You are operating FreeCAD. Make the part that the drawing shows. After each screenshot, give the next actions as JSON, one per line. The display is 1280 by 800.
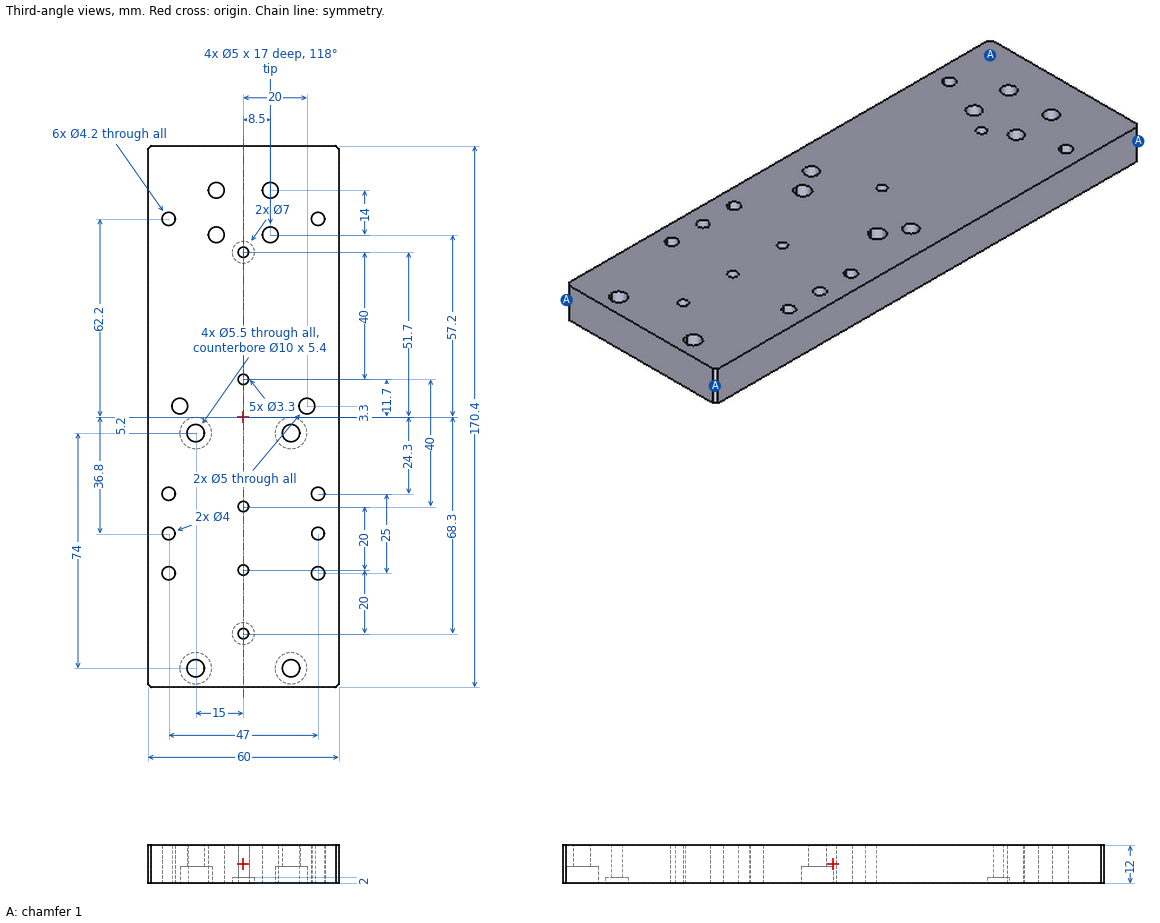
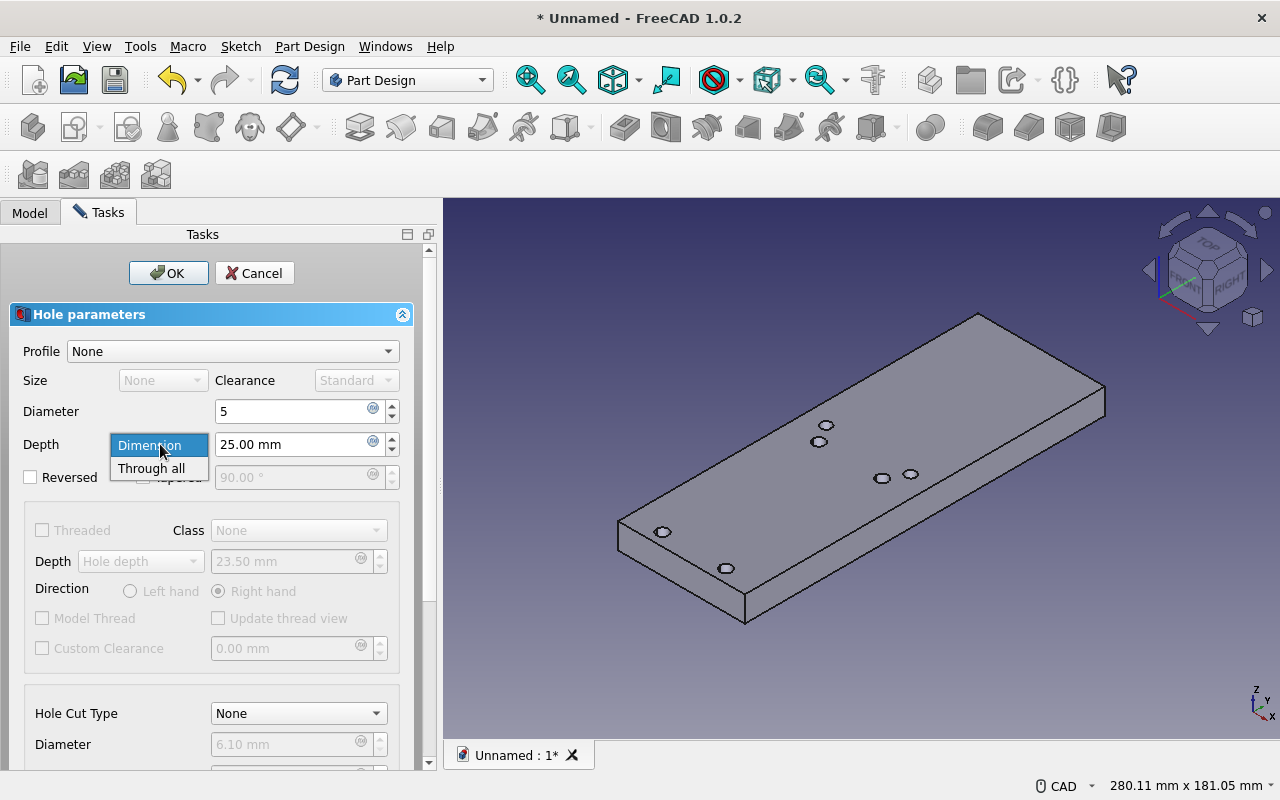
{"action": "left_click", "coordinate": [158, 468]}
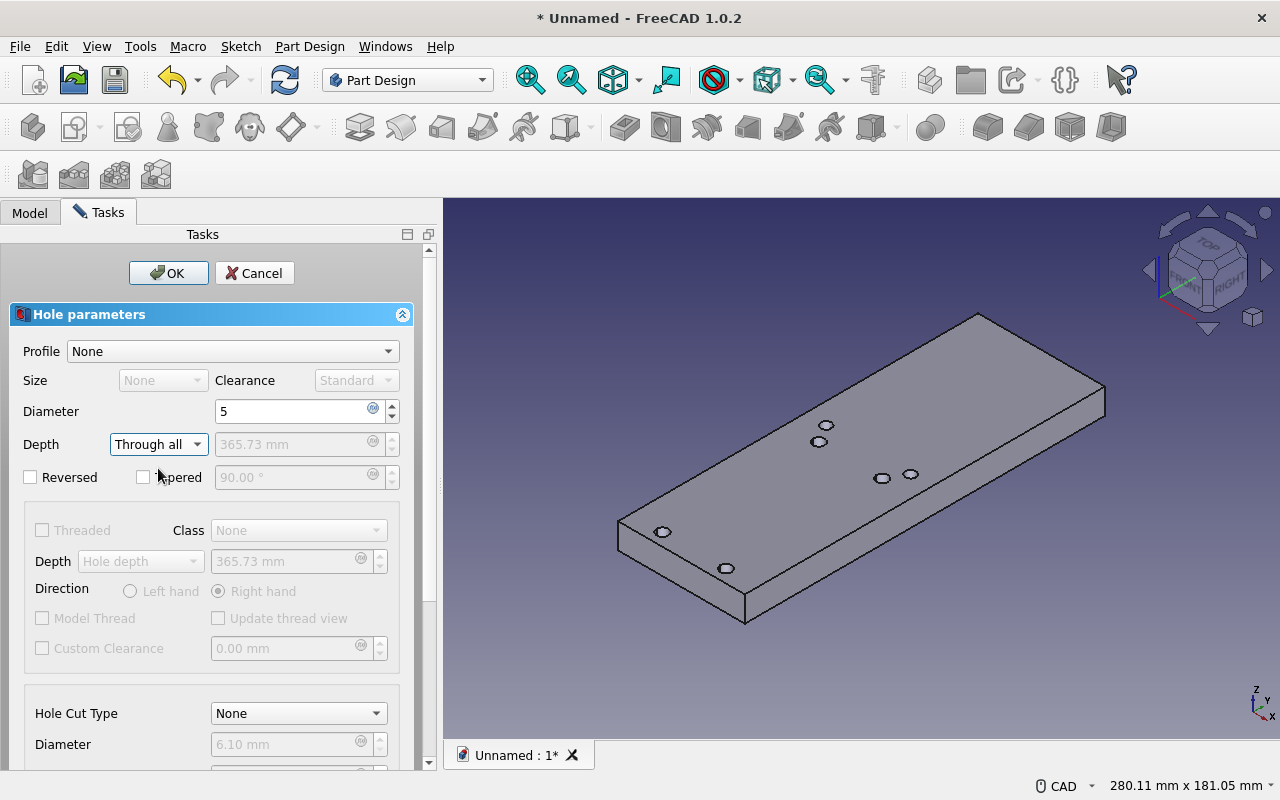
{"action": "left_click", "coordinate": [169, 273]}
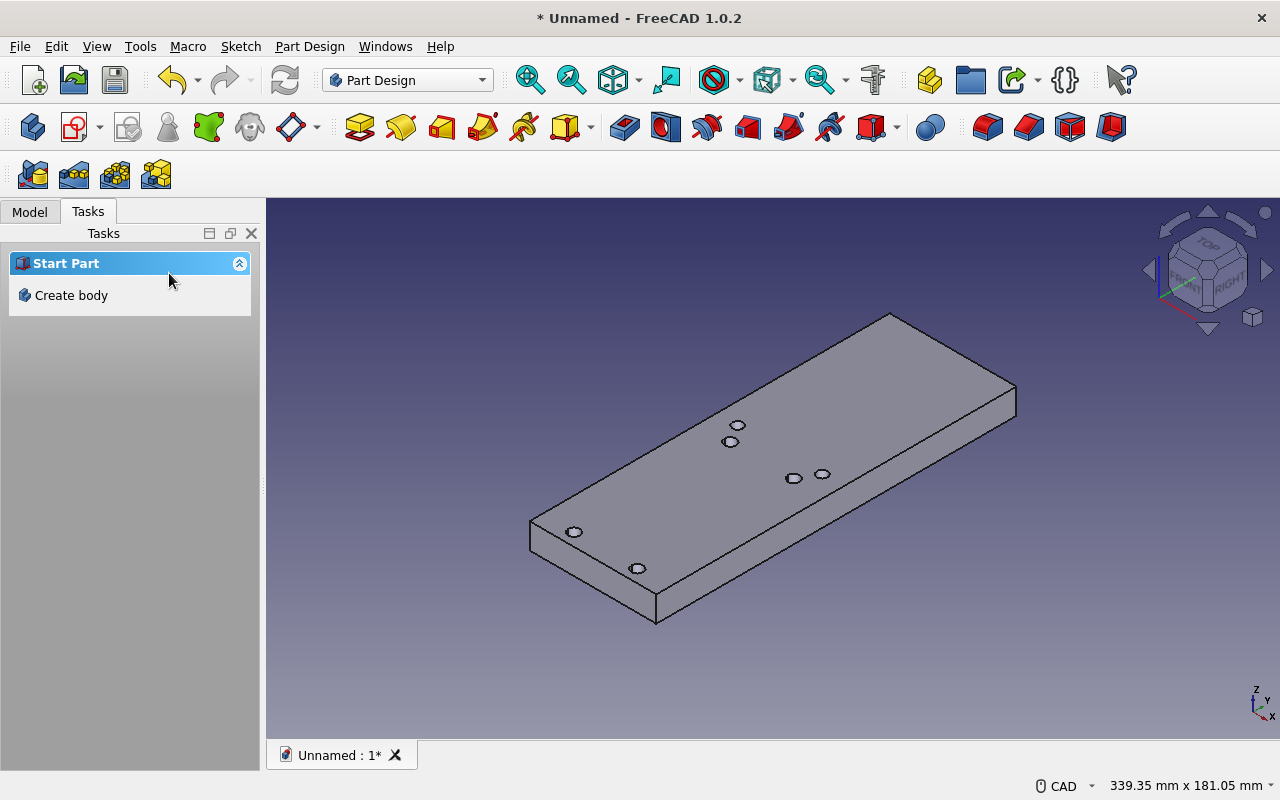
{"action": "key", "text": "5"}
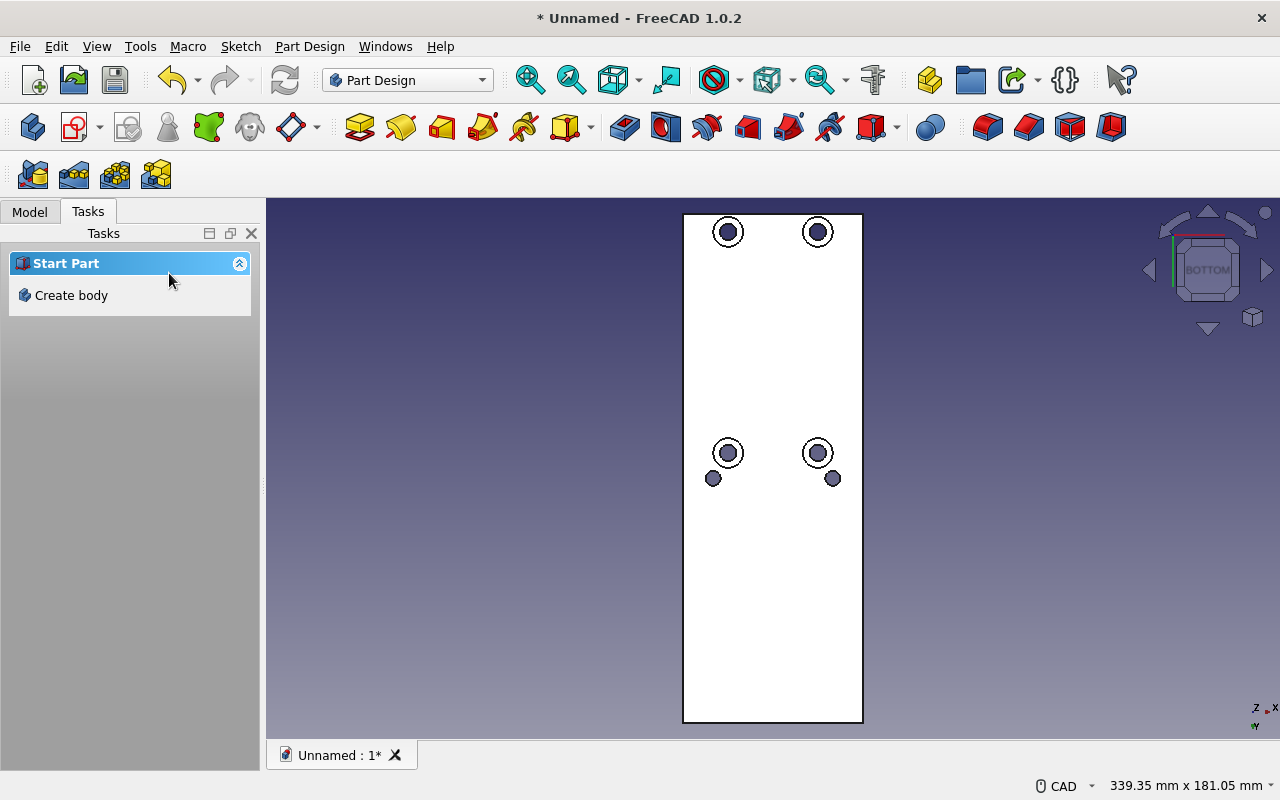
{"action": "left_click", "coordinate": [773, 613]}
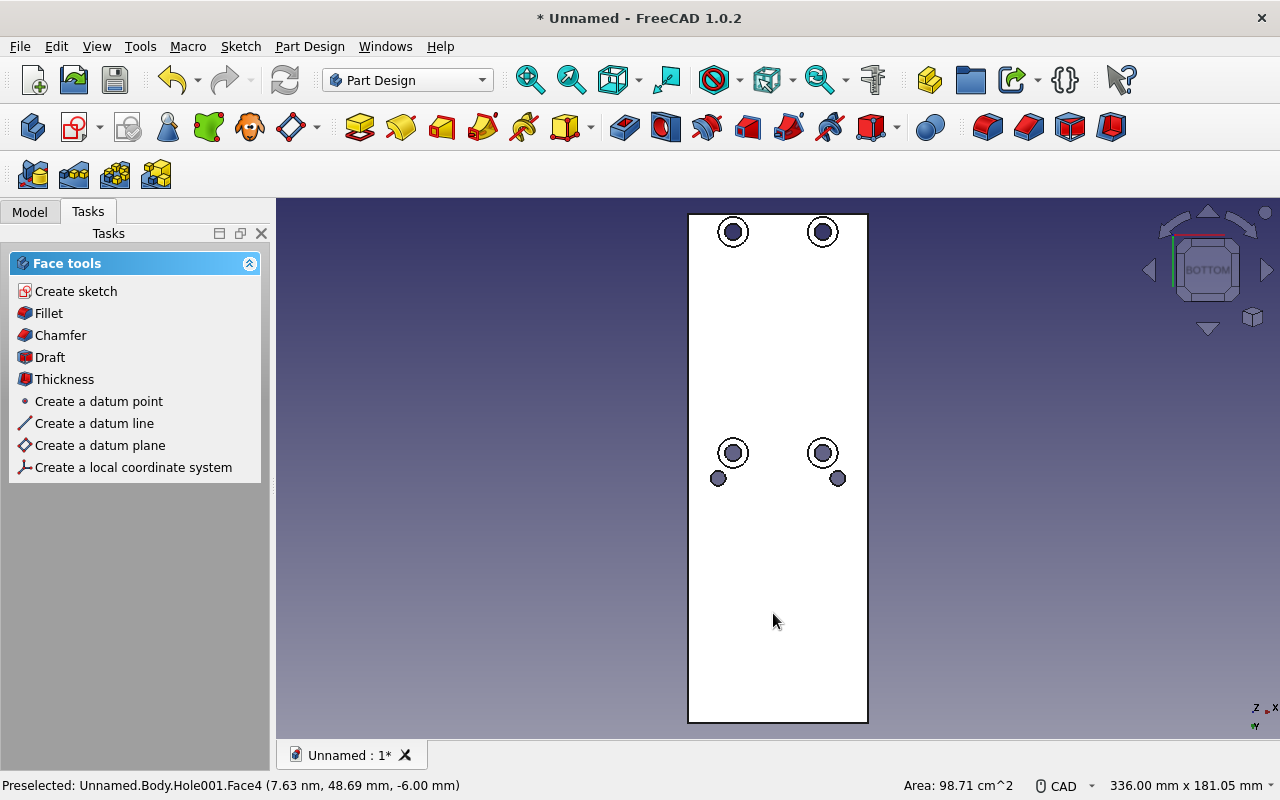
{"action": "left_click", "coordinate": [74, 128]}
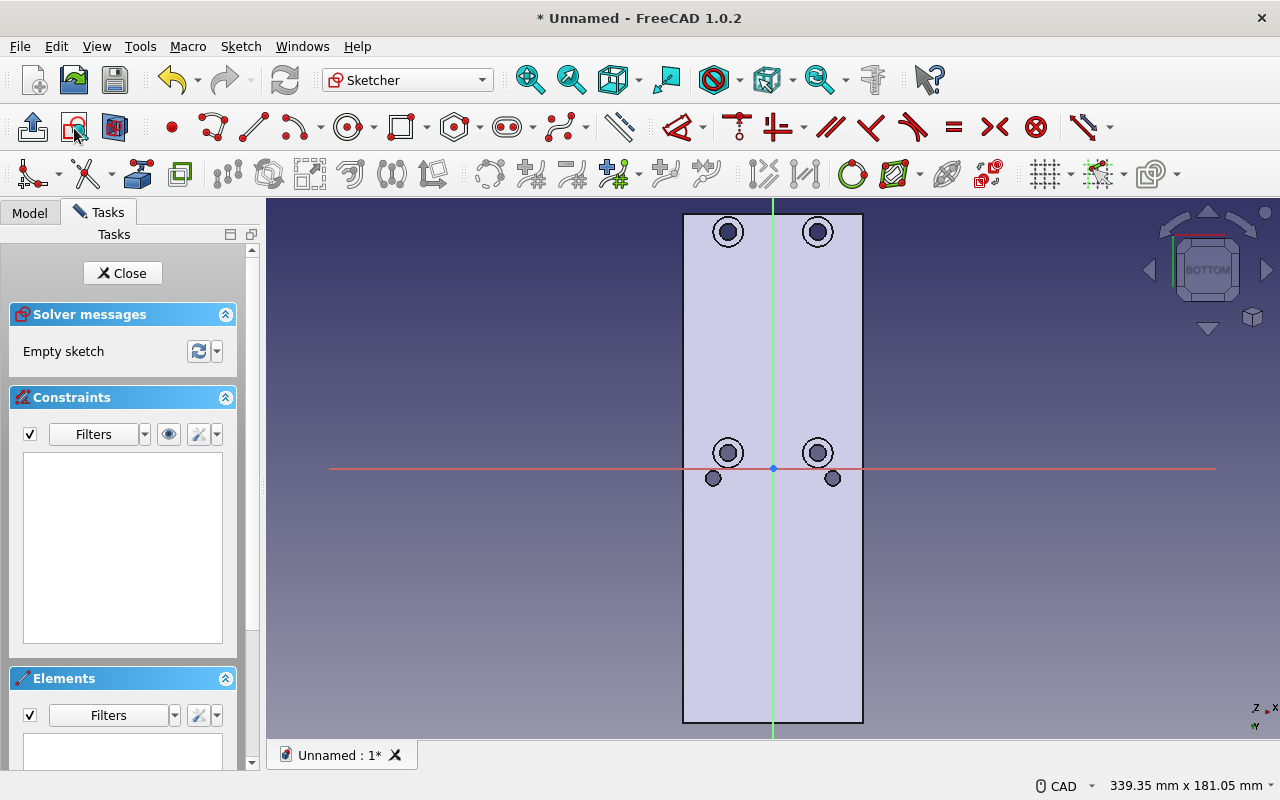
{"action": "left_click", "coordinate": [348, 128]}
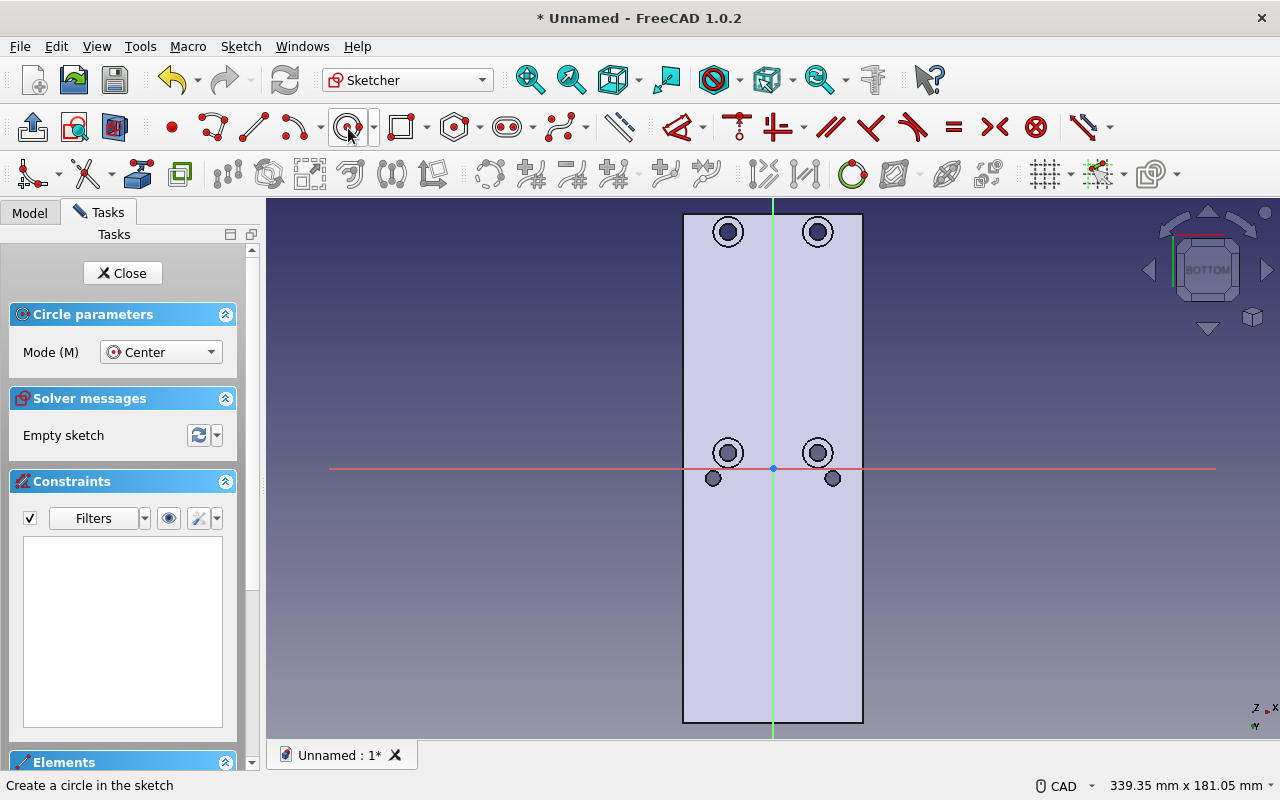
{"action": "scroll", "coordinate": [773, 503], "scroll_direction": "up", "scroll_amount": 8}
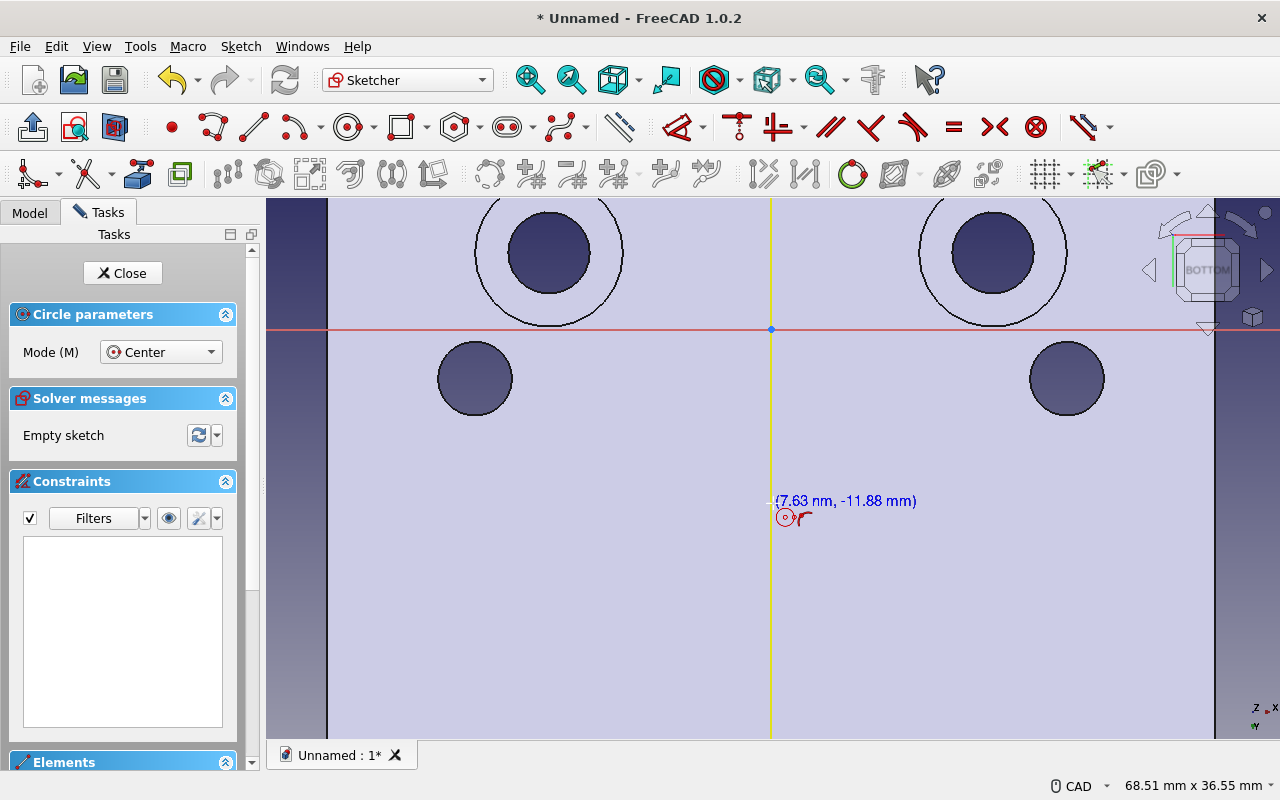
{"action": "scroll", "coordinate": [688, 535], "scroll_direction": "down", "scroll_amount": 8}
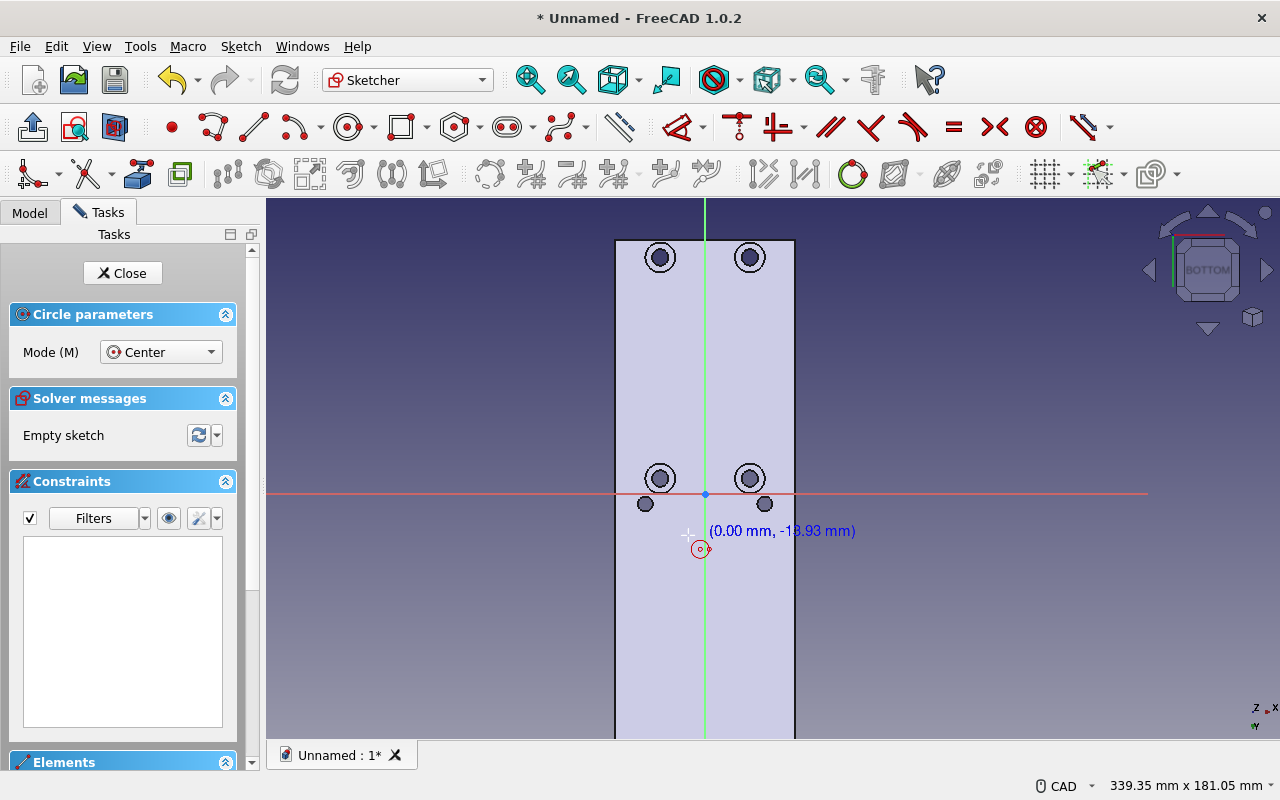
{"action": "left_click", "coordinate": [705, 529]}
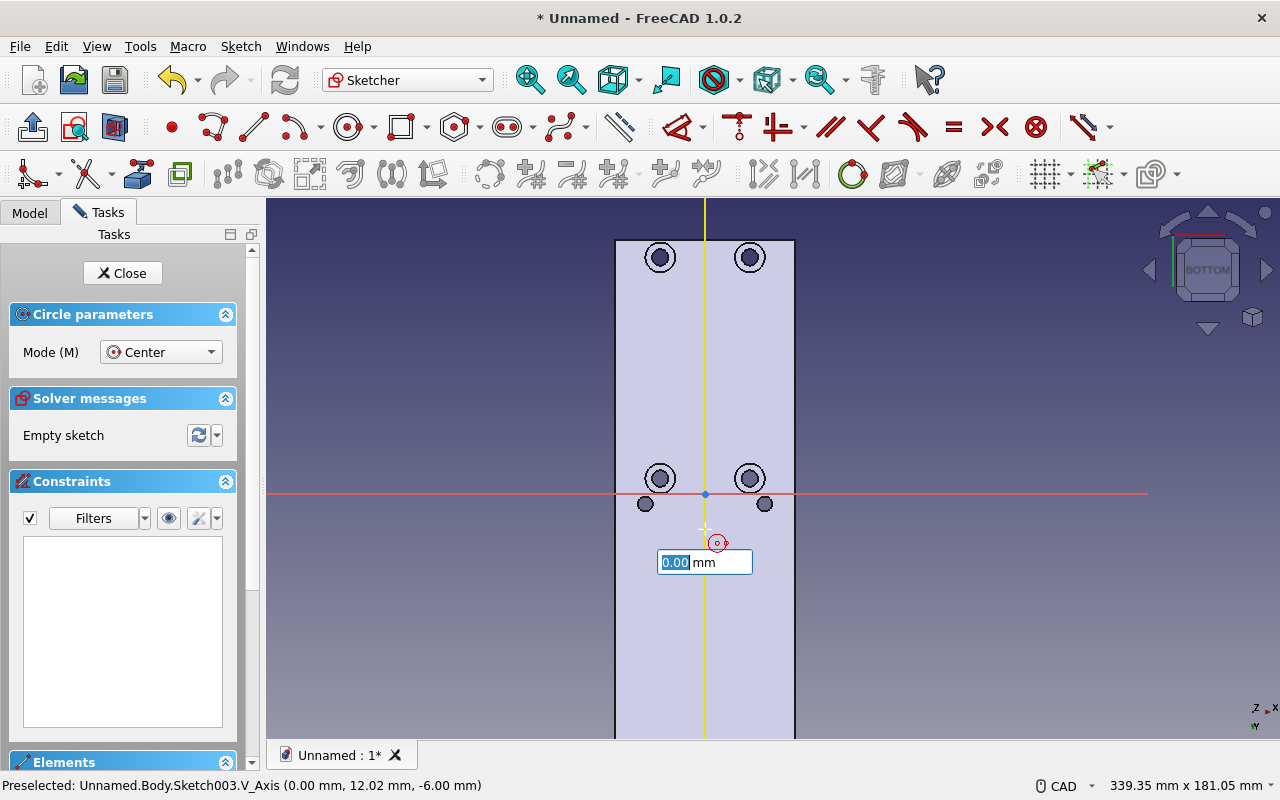
{"action": "scroll", "coordinate": [710, 527], "scroll_direction": "up", "scroll_amount": 7}